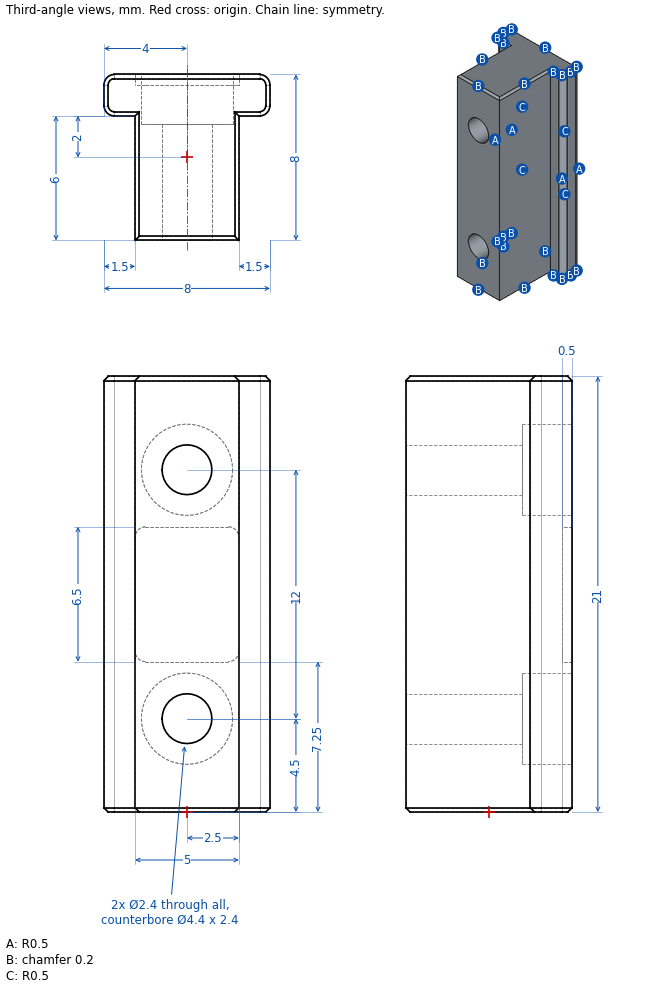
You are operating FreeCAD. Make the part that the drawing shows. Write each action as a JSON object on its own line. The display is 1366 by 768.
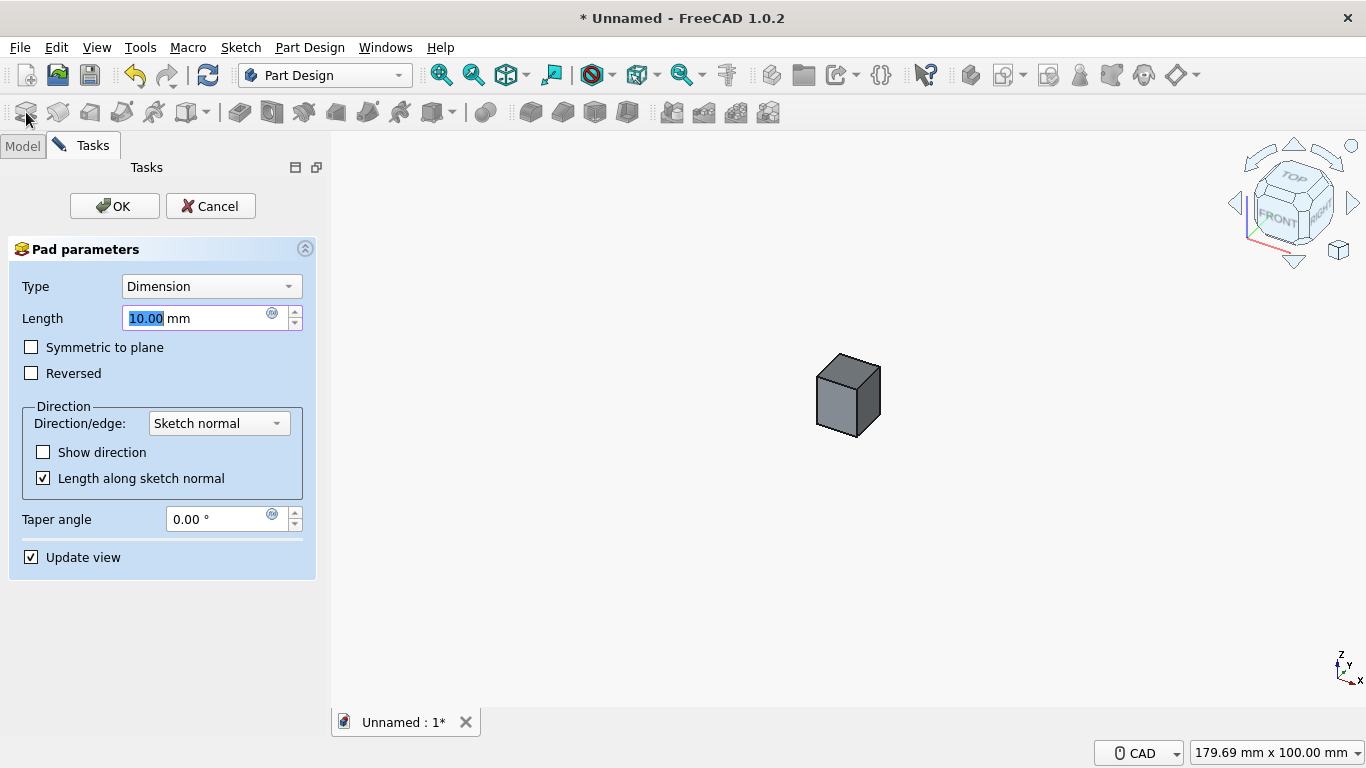
{"action": "type", "text": "21"}
{"action": "key", "text": "Tab"}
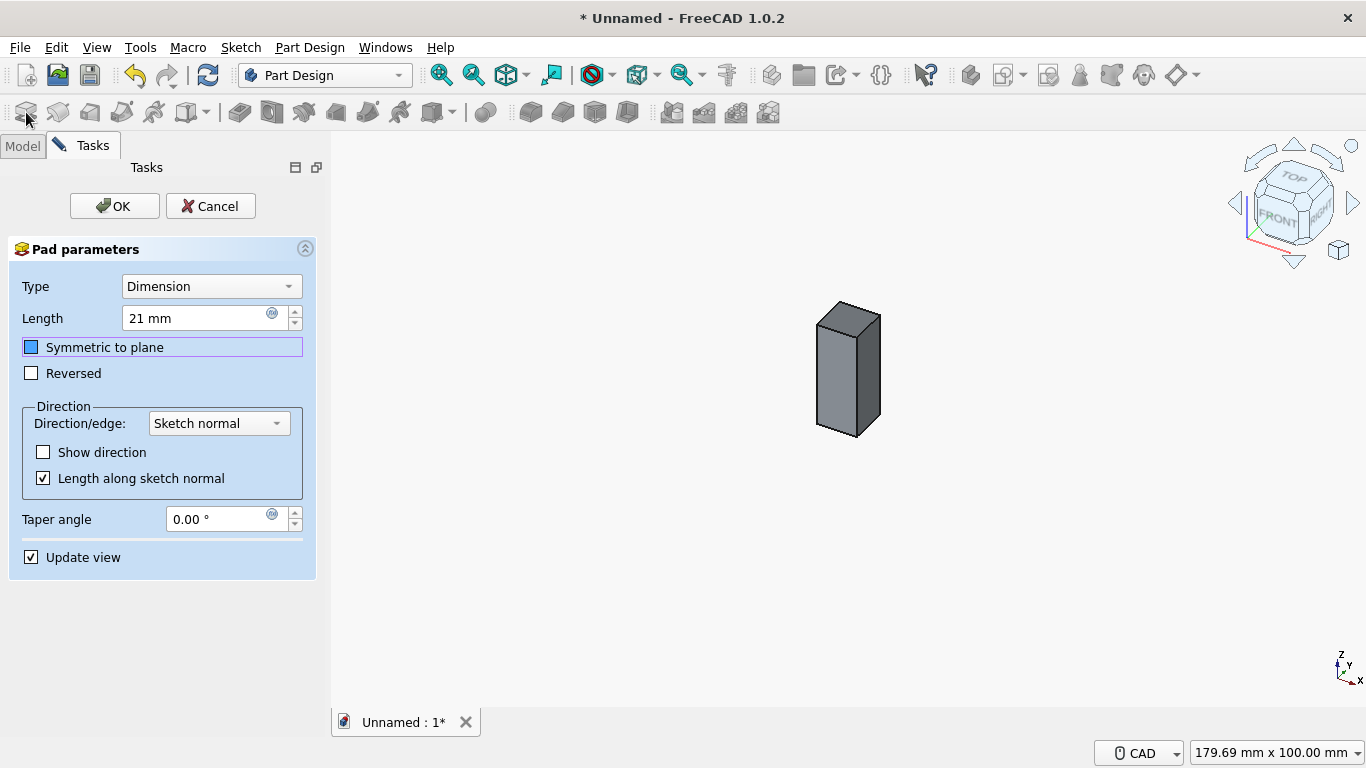
{"action": "left_click", "coordinate": [115, 206]}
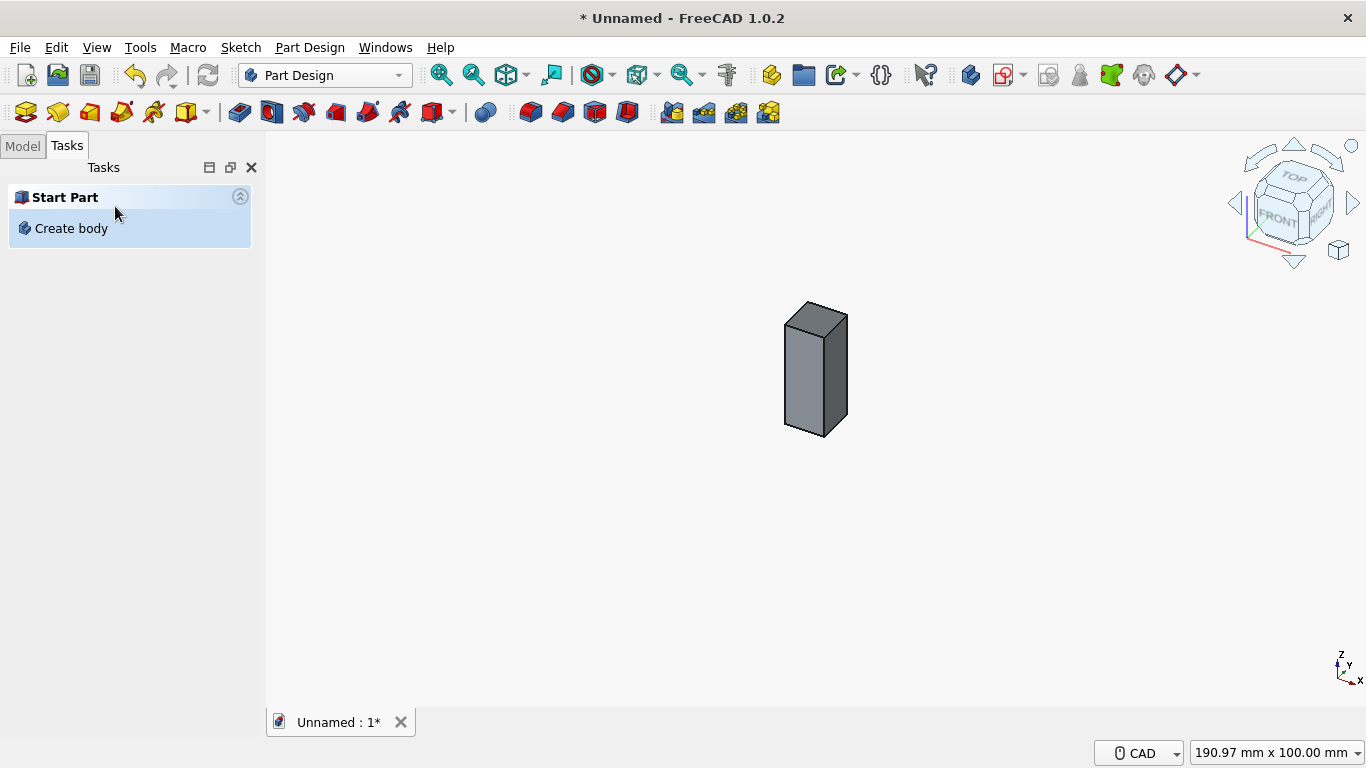
{"action": "left_click", "coordinate": [442, 76]}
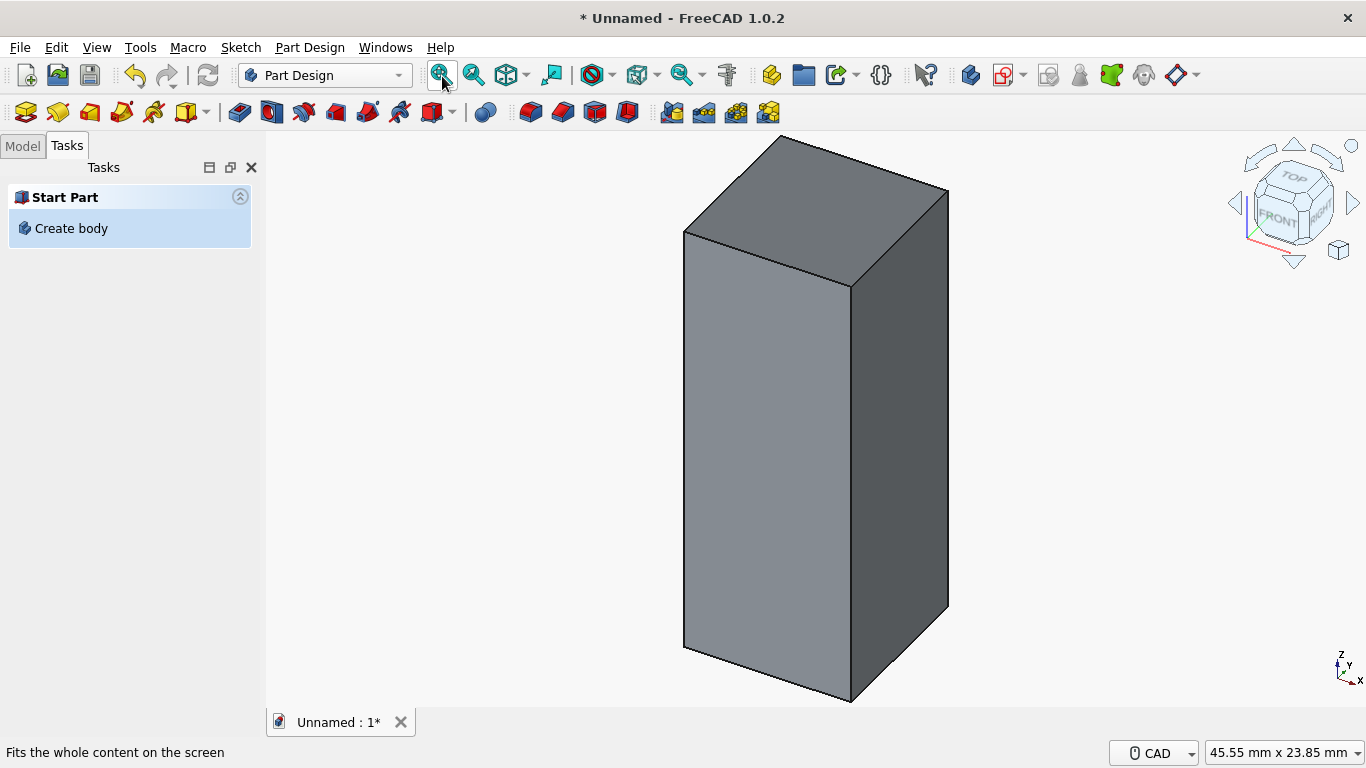
{"action": "left_click", "coordinate": [816, 210]}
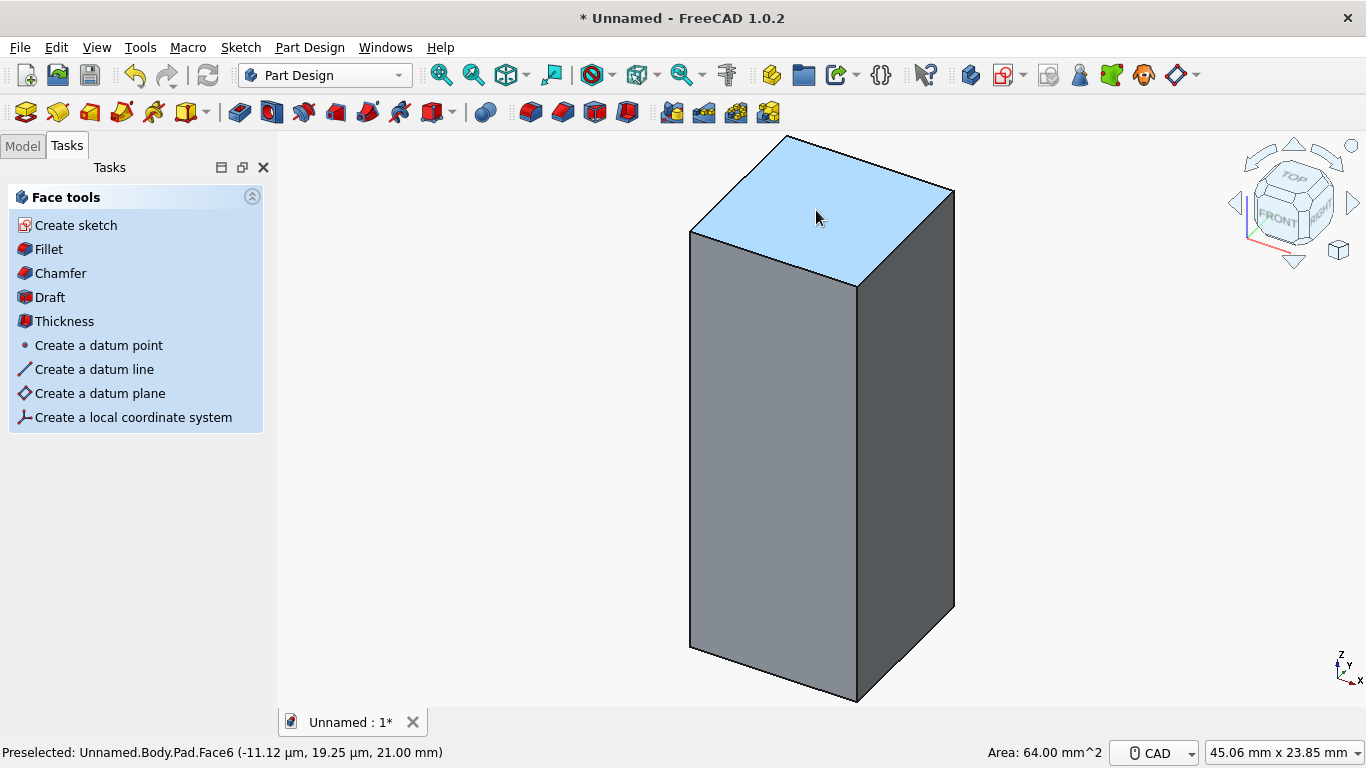
{"action": "left_click", "coordinate": [1004, 76]}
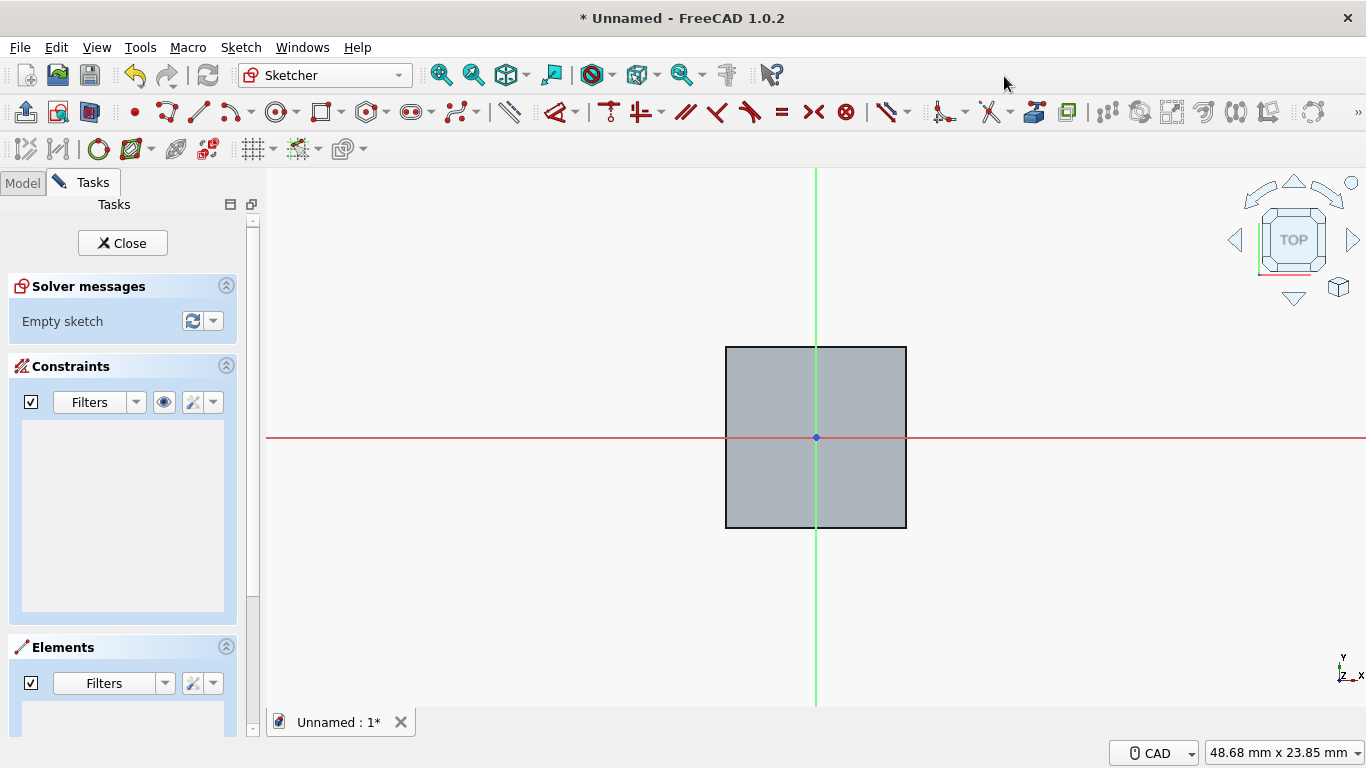
{"action": "scroll", "coordinate": [856, 473], "scroll_direction": "up", "scroll_amount": 5}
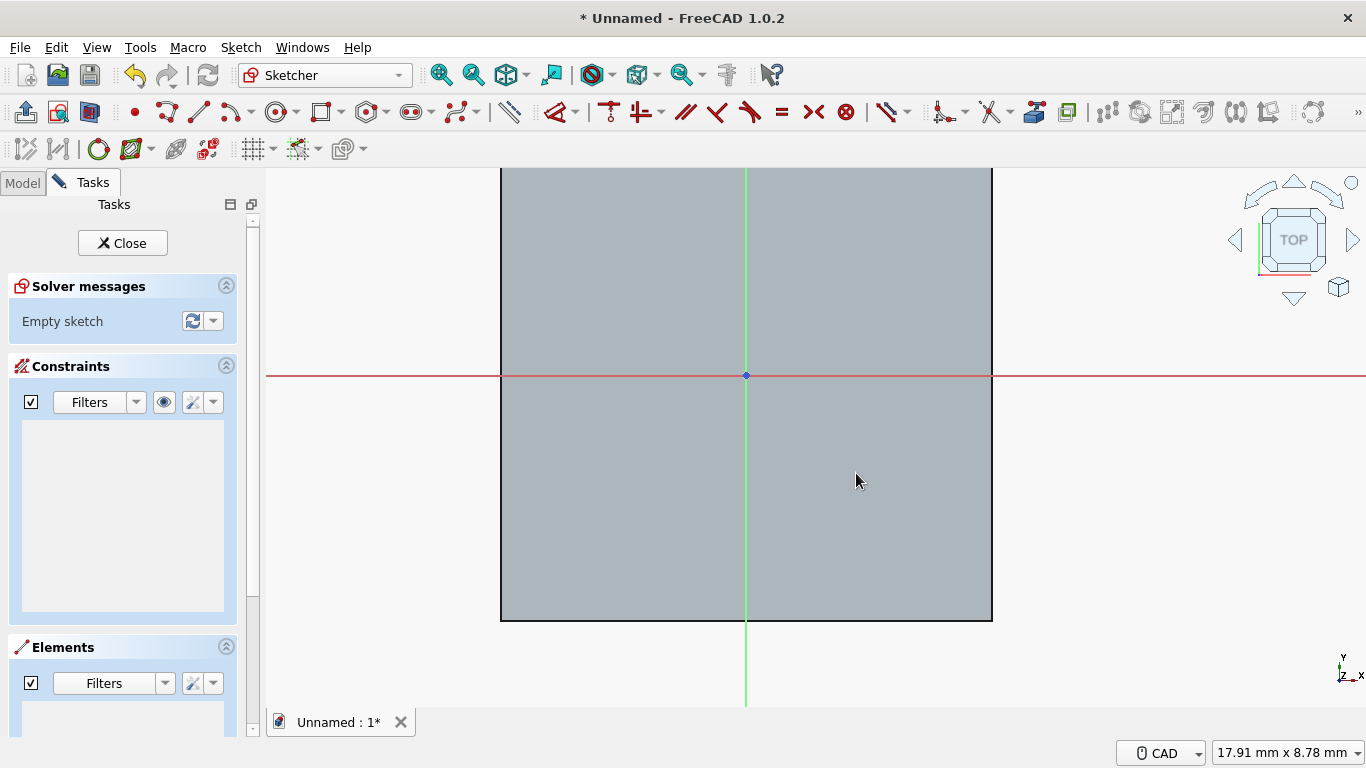
{"action": "left_click", "coordinate": [322, 112]}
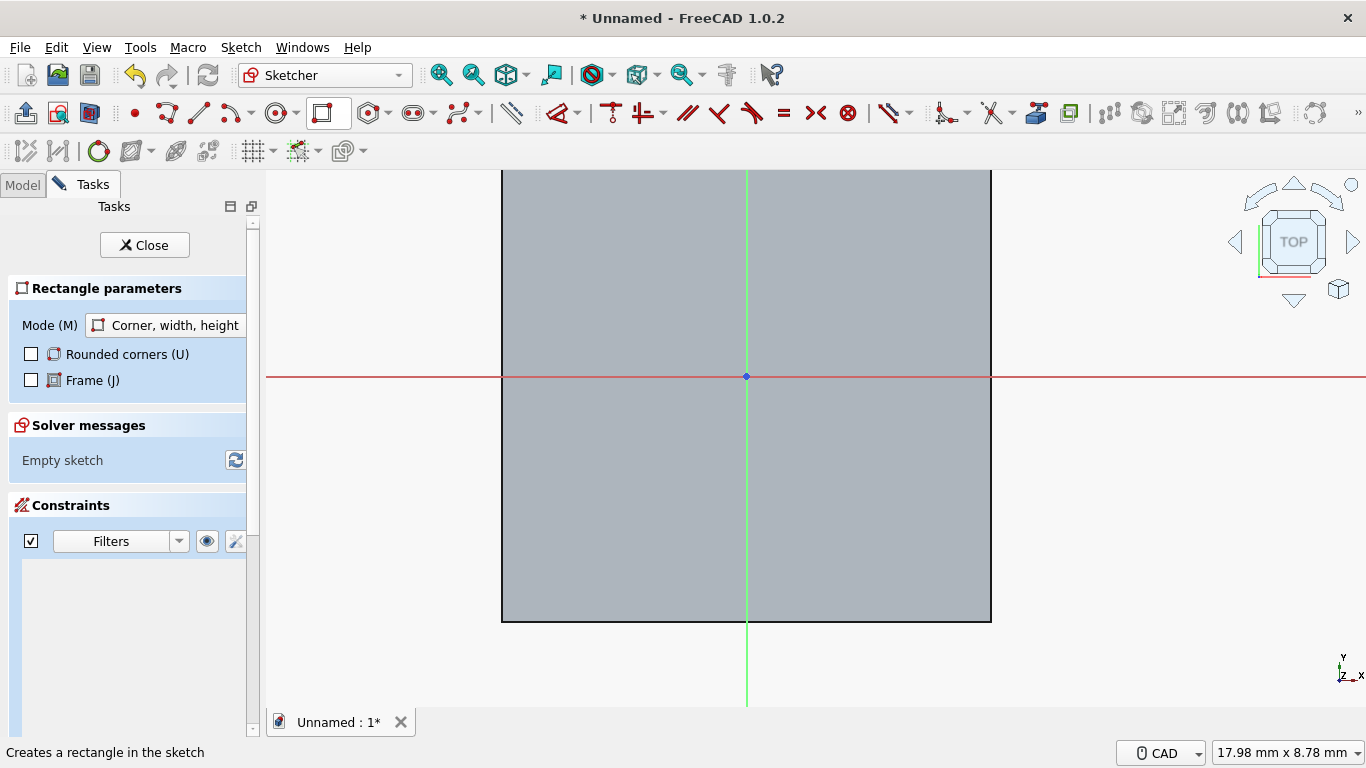
{"action": "left_click", "coordinate": [502, 254]}
{"action": "mouse_move", "coordinate": [594, 622]}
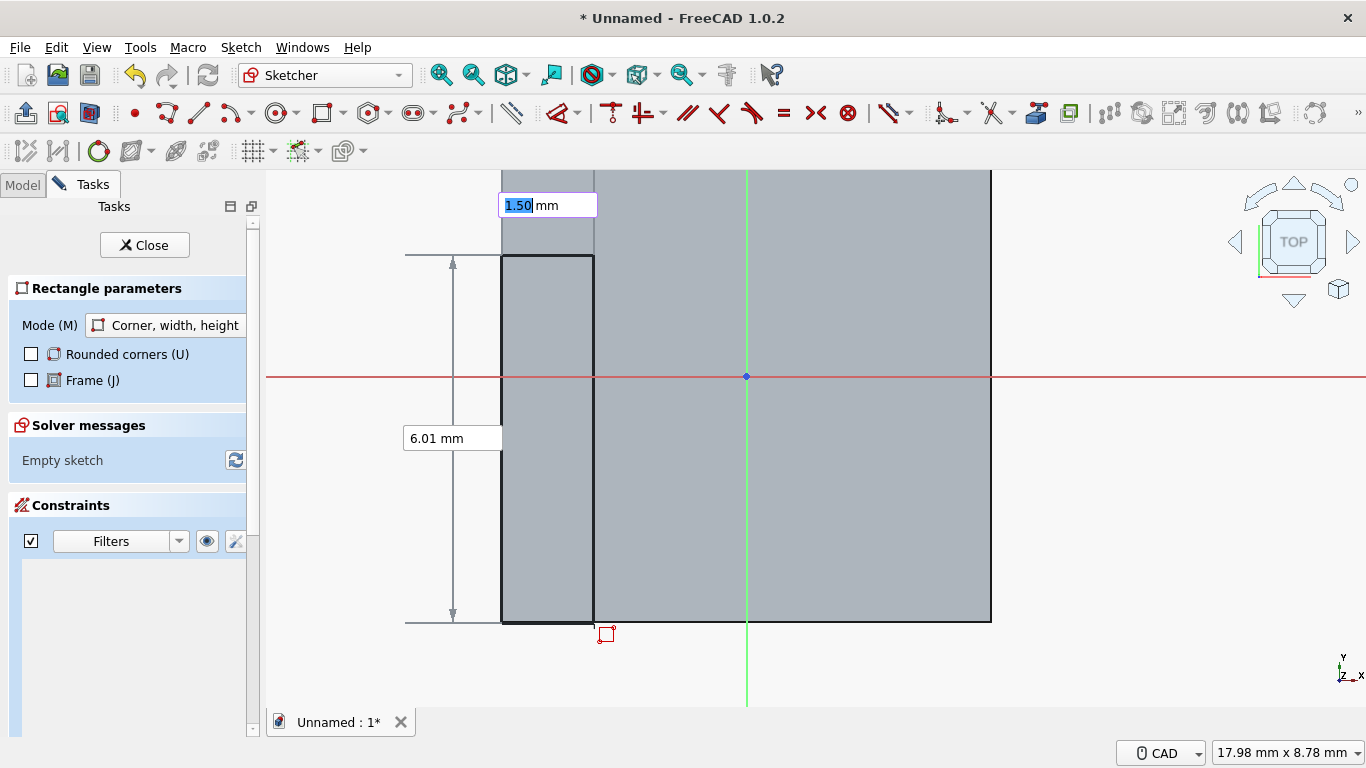
{"action": "type", "text": "1.5"}
{"action": "key", "text": "Tab"}
{"action": "type", "text": "6"}
{"action": "key", "text": "Return"}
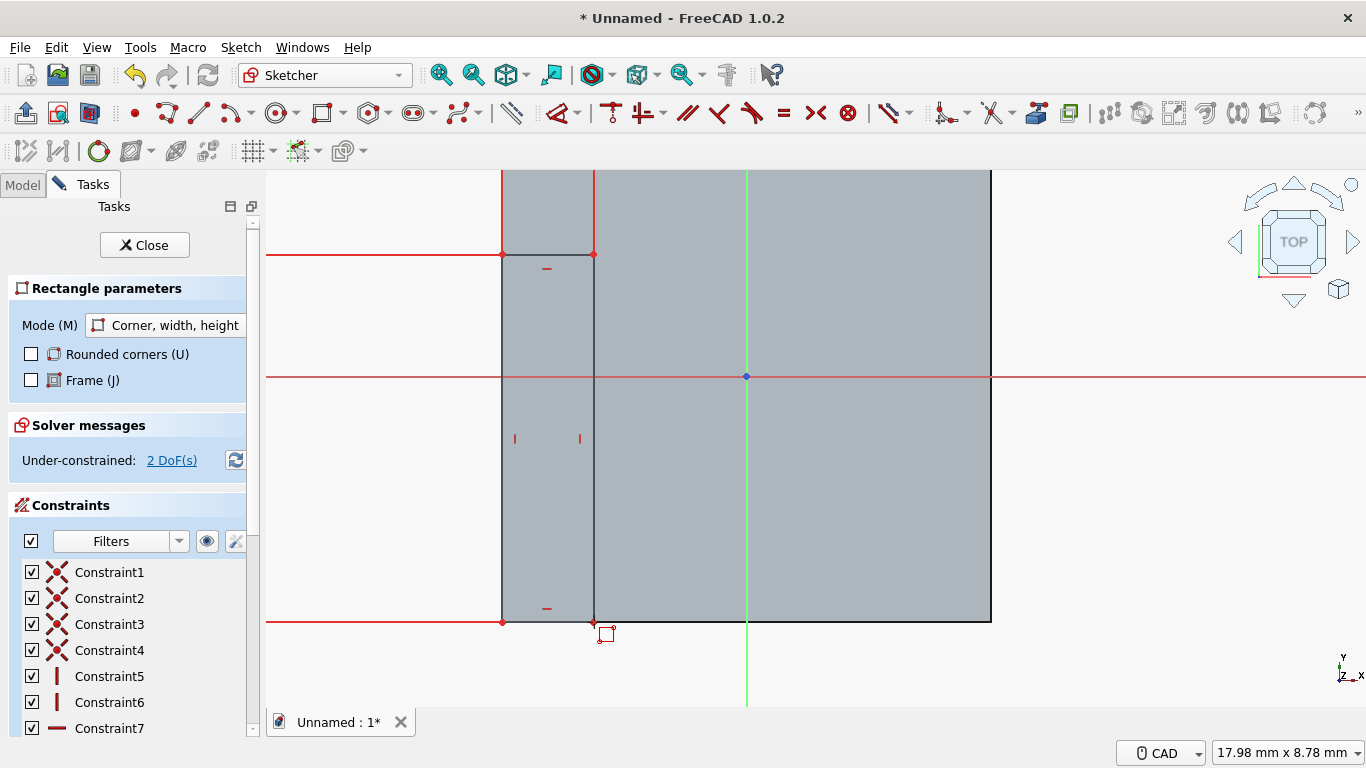
{"action": "left_click", "coordinate": [900, 254]}
{"action": "mouse_move", "coordinate": [991, 622]}